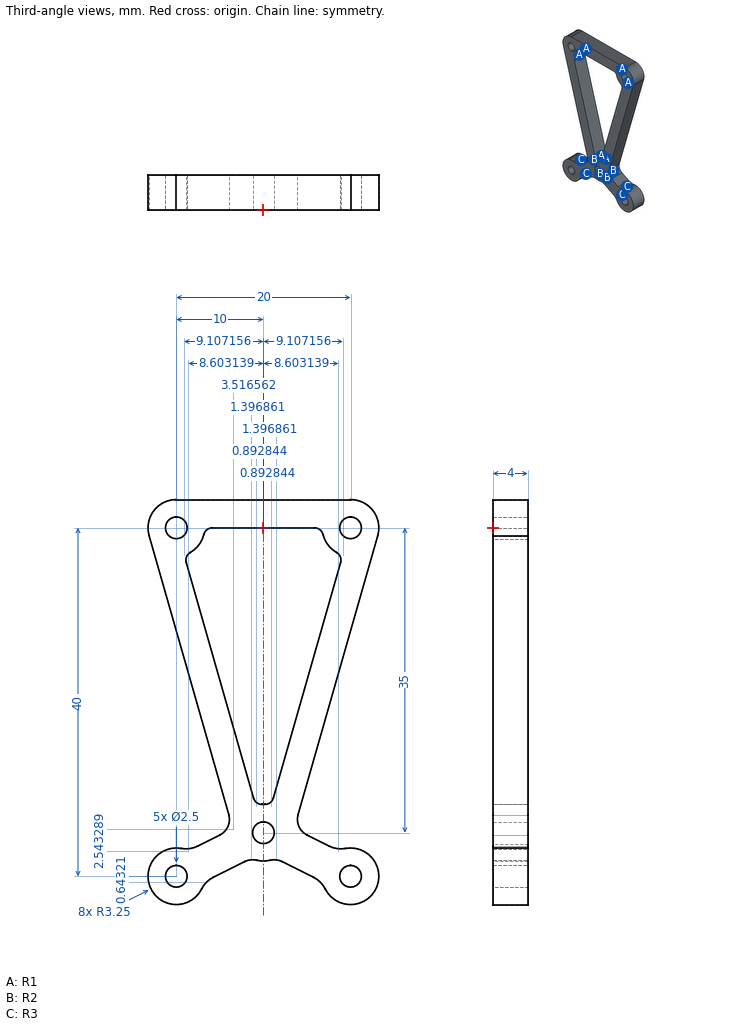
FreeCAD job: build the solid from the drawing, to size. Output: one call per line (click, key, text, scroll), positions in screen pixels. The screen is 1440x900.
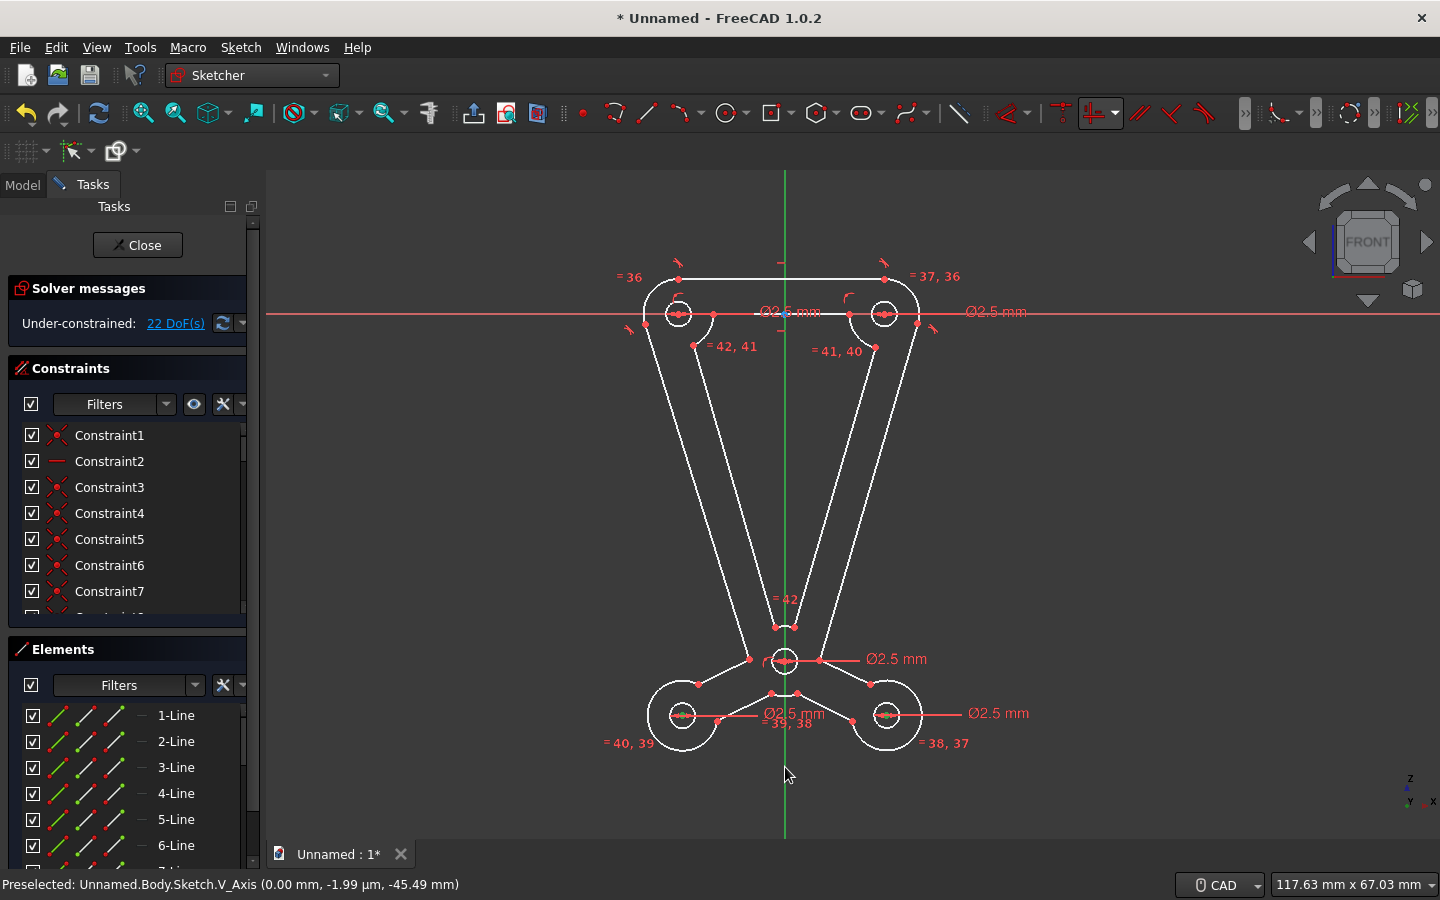
key(s)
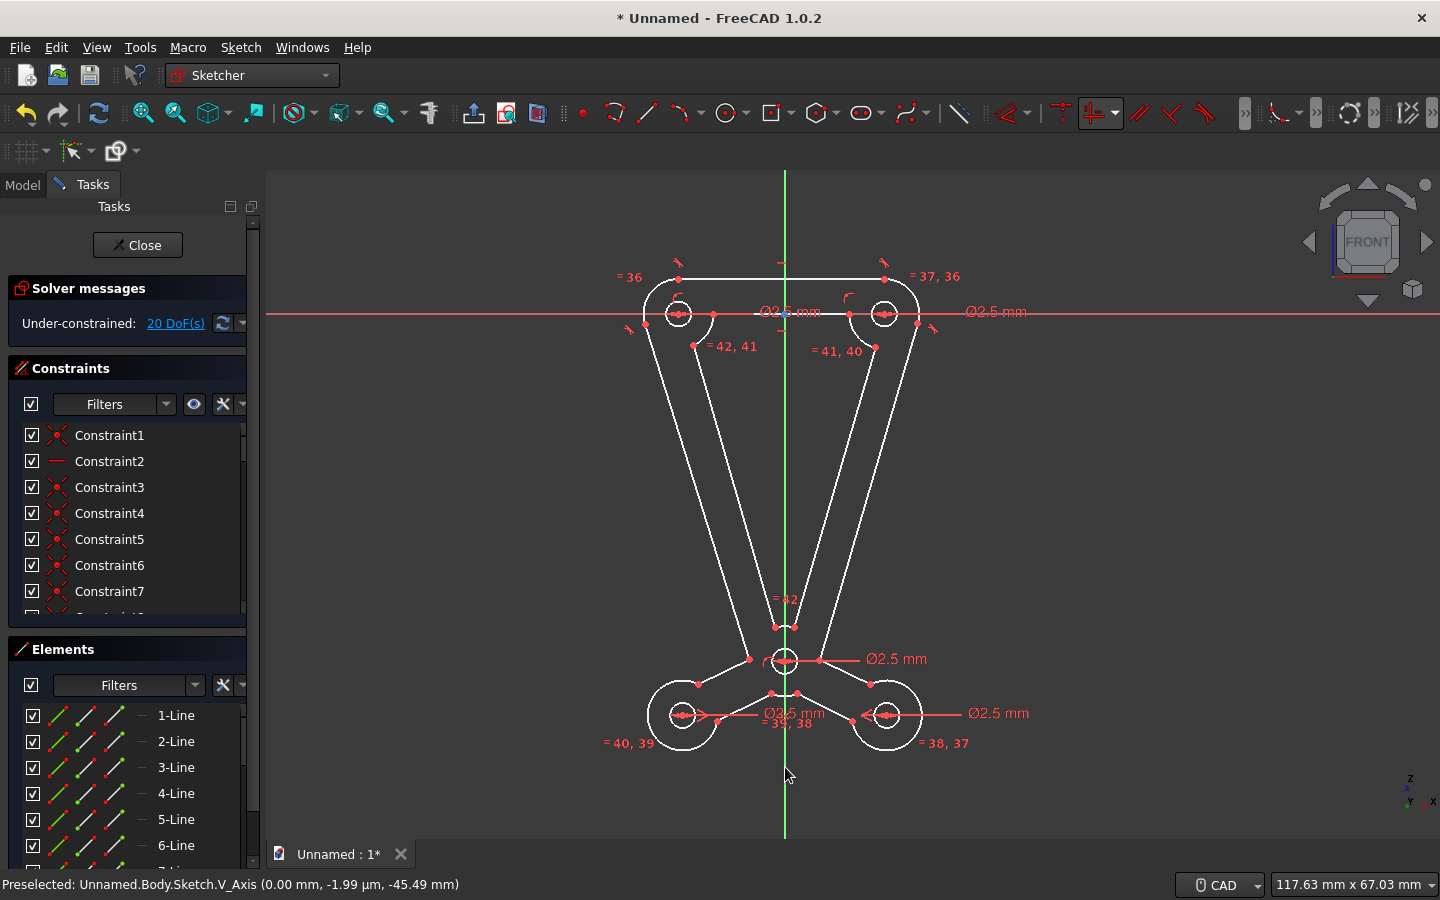
click(749, 660)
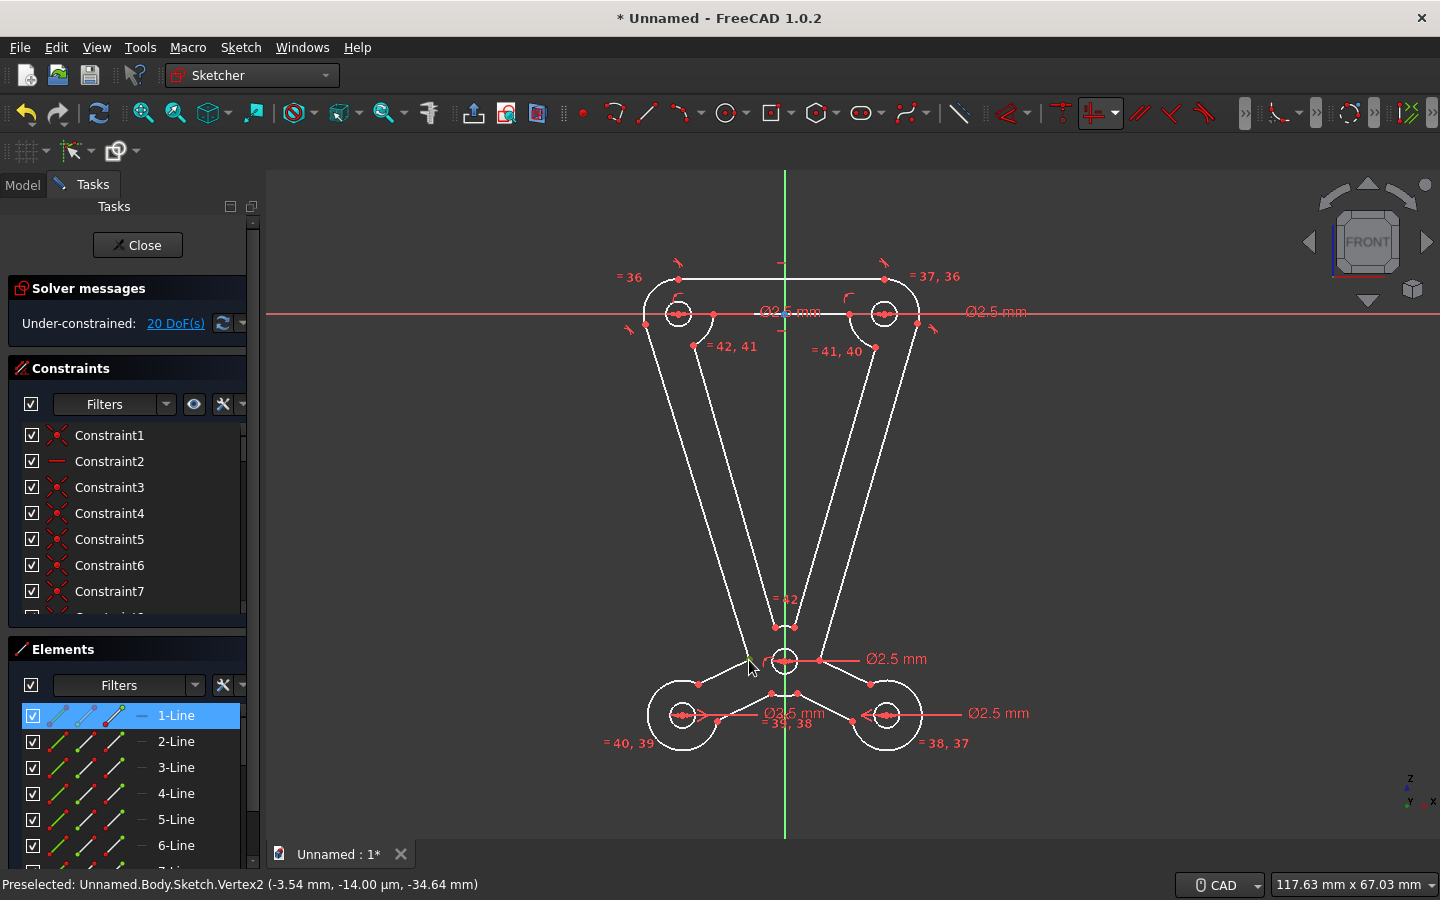
click(820, 660)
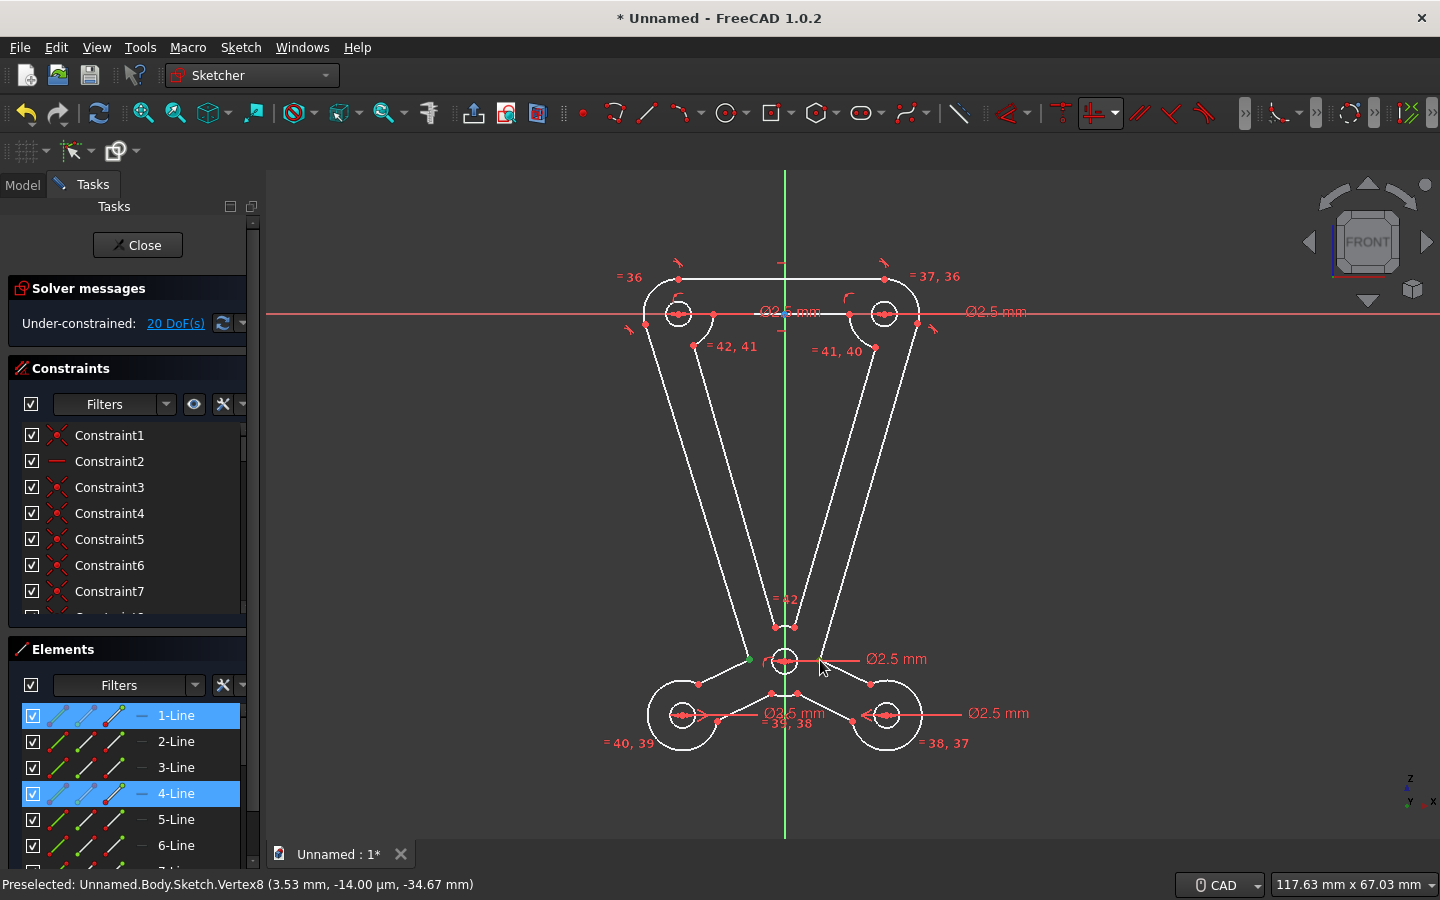
click(785, 767)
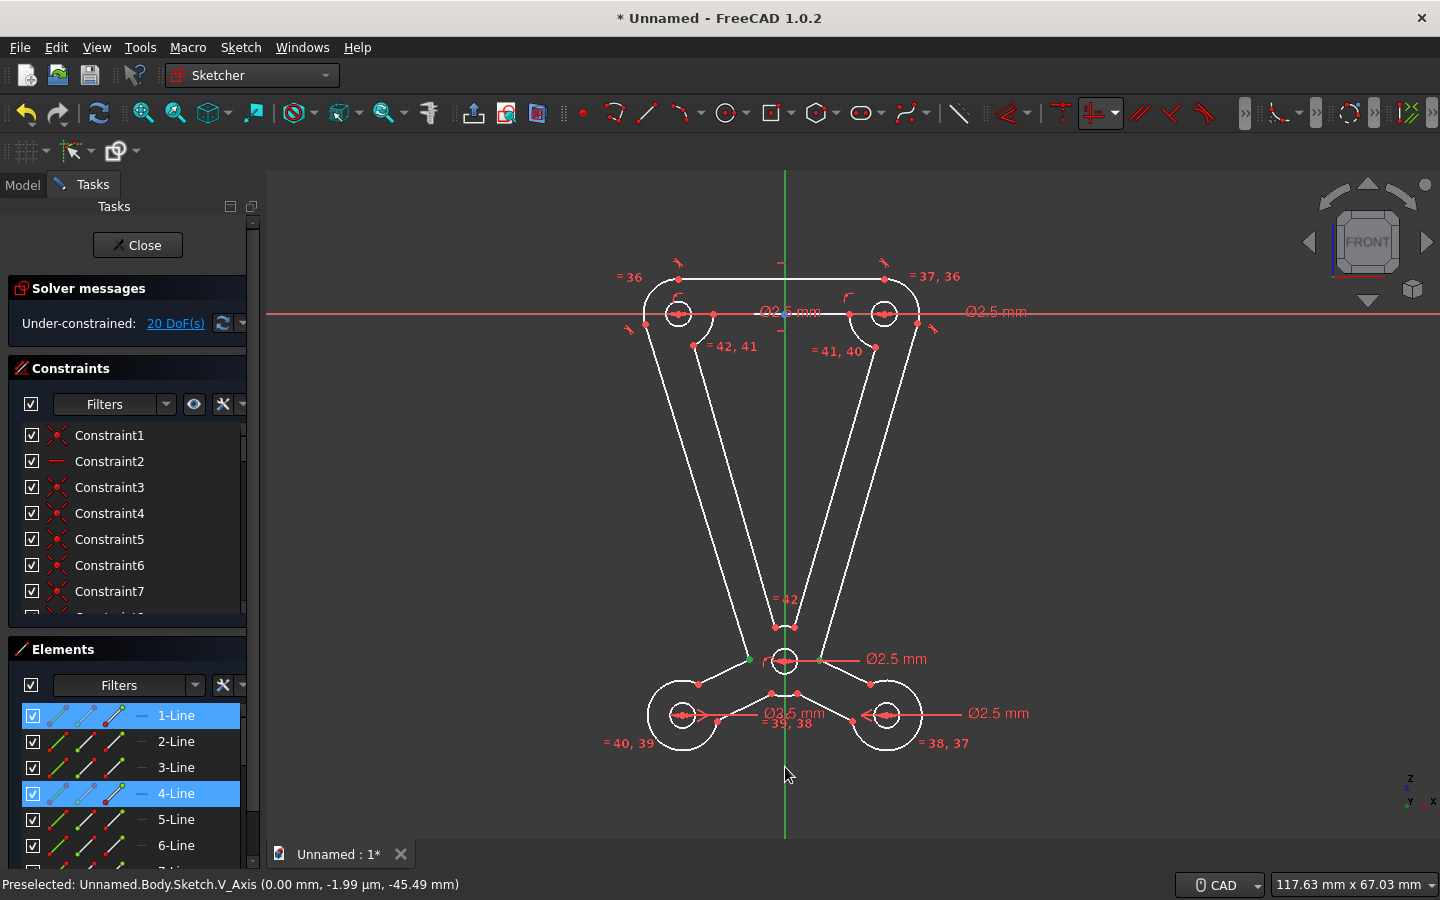
key(s)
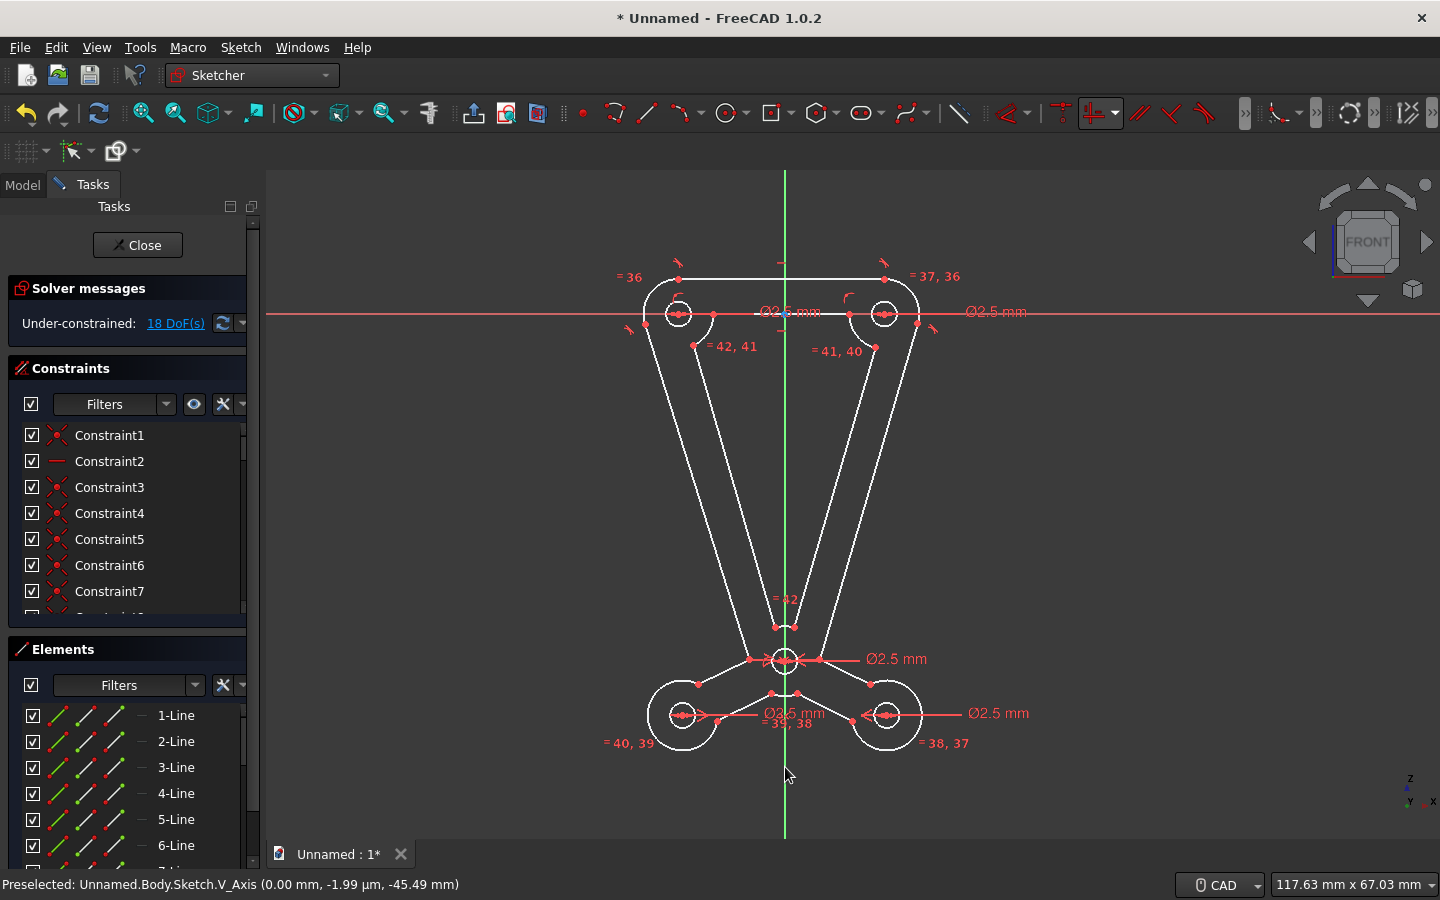
click(1006, 114)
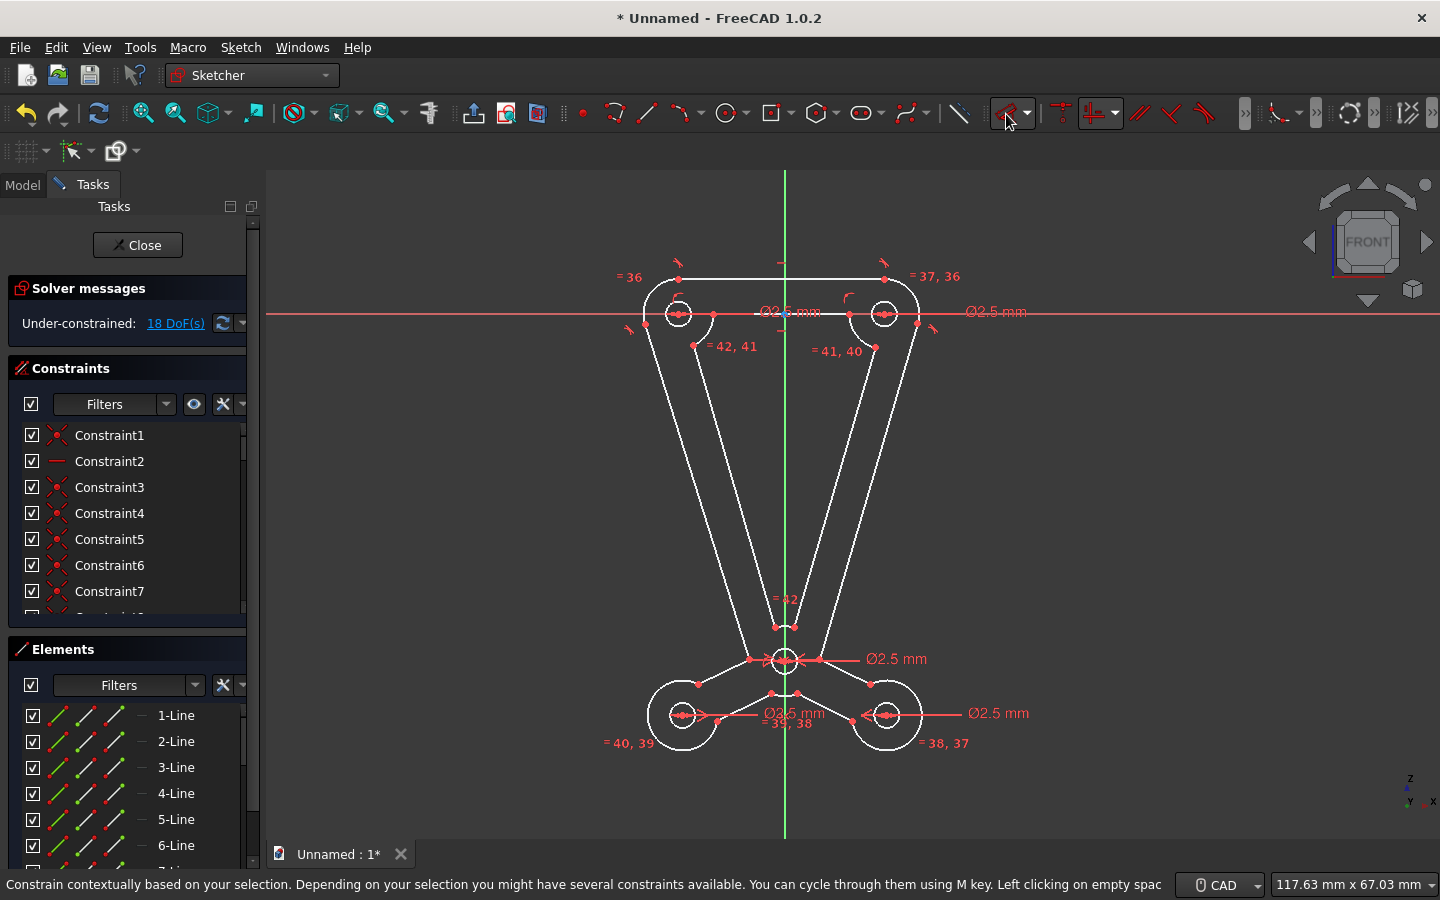
scroll(660, 284, up, 2)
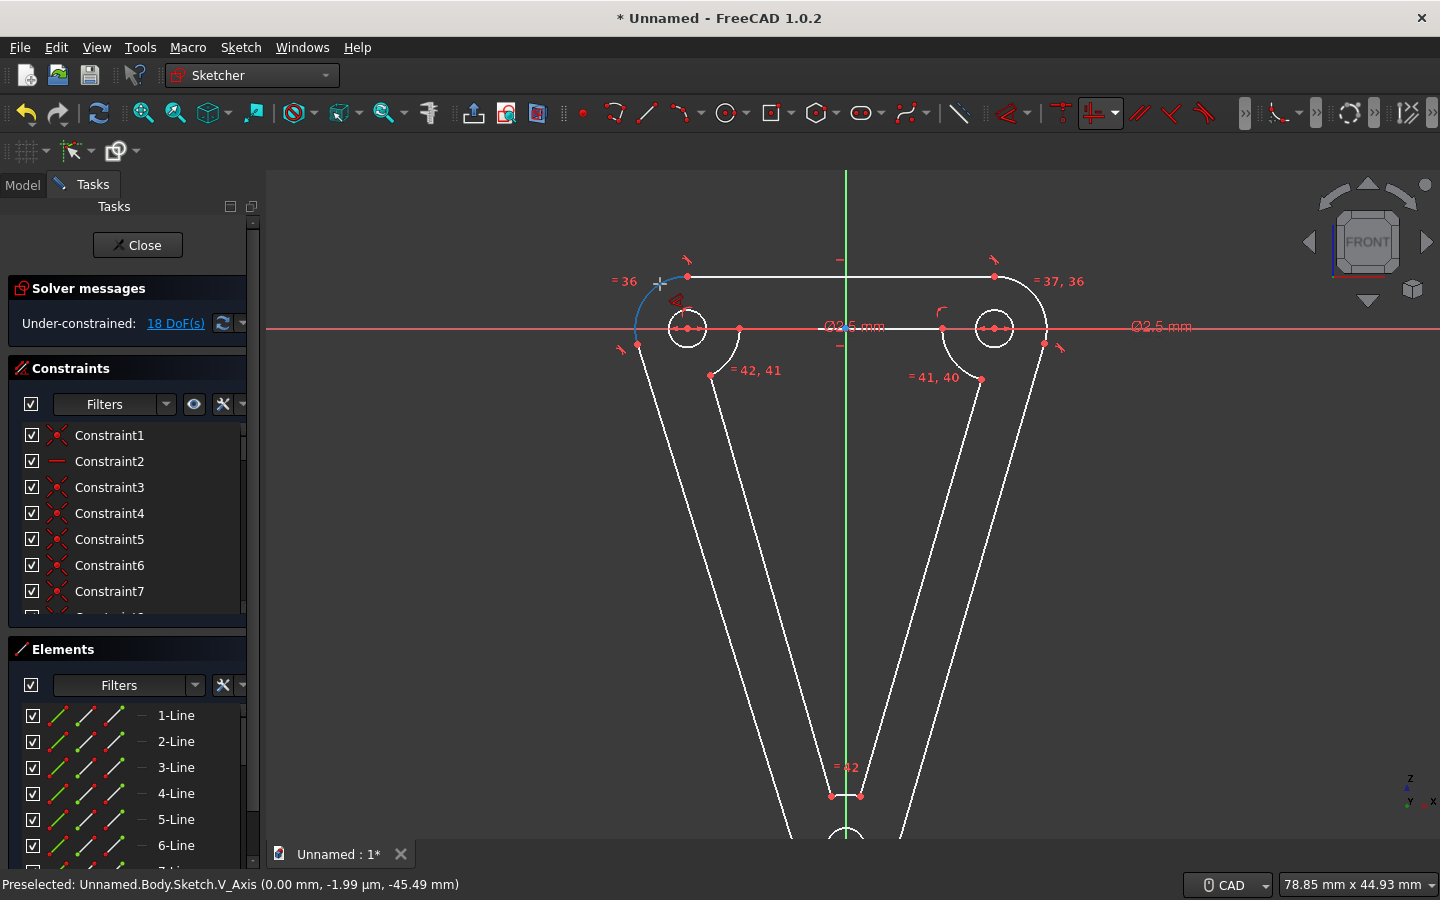
click(660, 285)
click(643, 258)